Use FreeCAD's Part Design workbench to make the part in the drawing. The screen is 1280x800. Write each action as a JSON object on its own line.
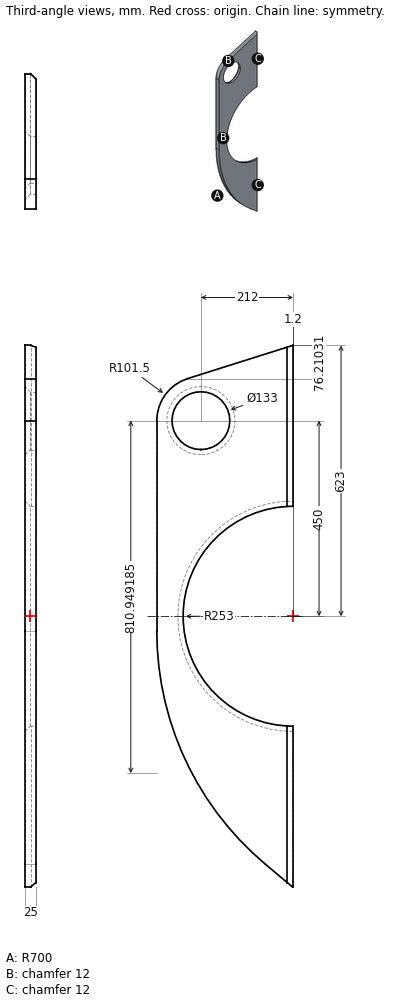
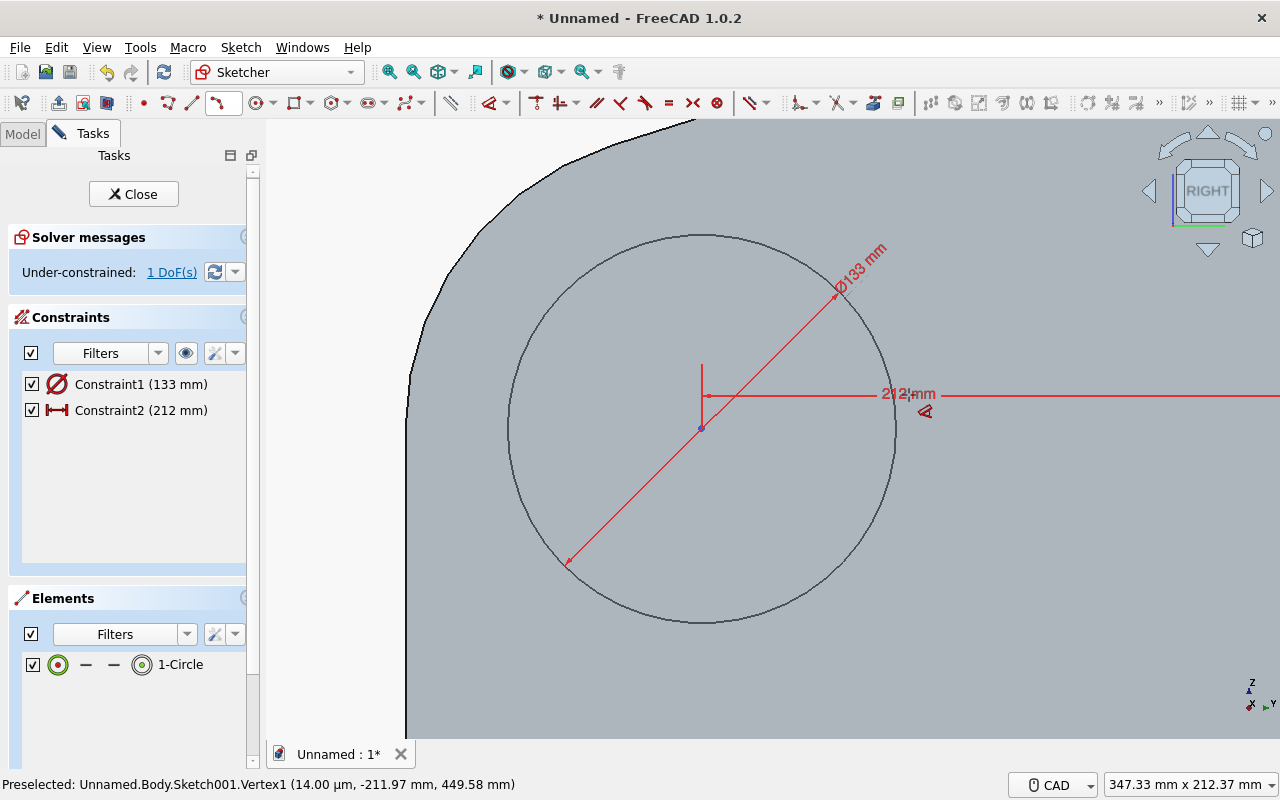
{"action": "left_click", "coordinate": [702, 429]}
{"action": "left_click", "coordinate": [668, 570]}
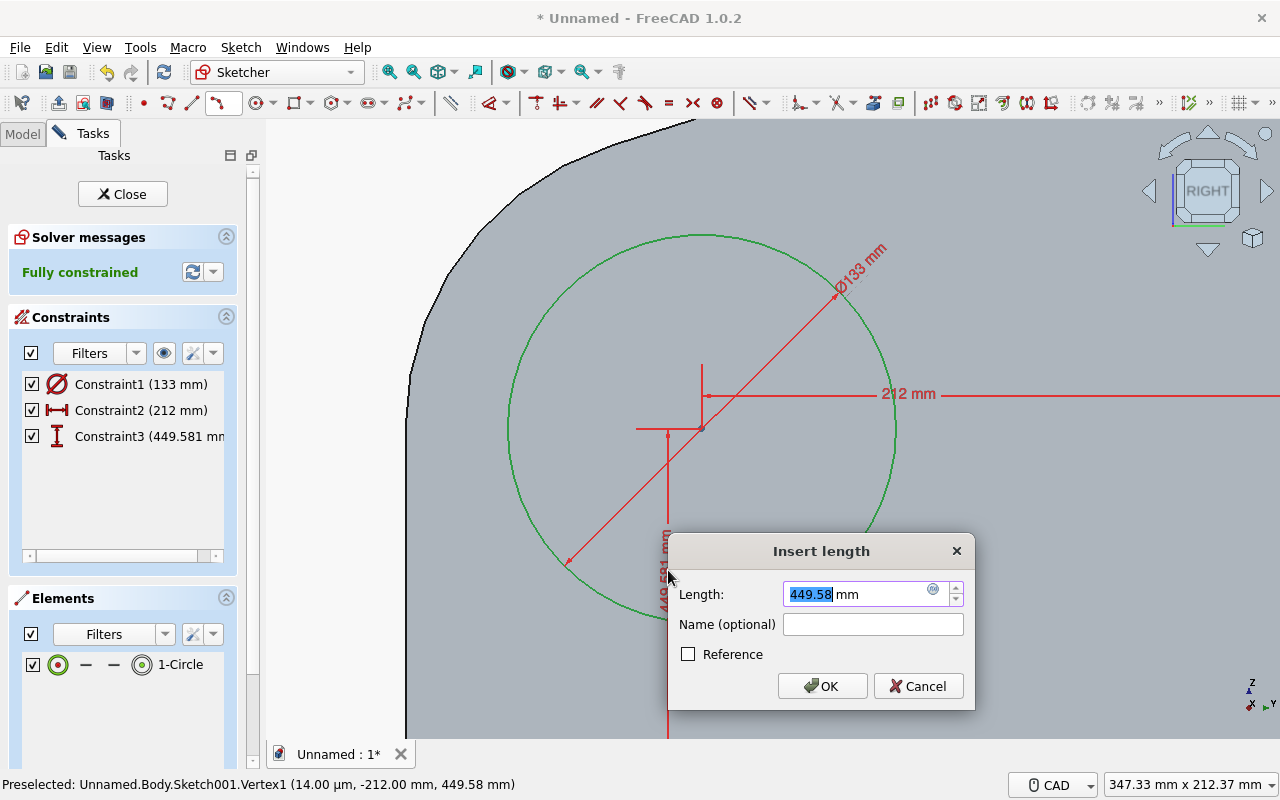
{"action": "type", "text": "450"}
{"action": "key", "text": "Return"}
{"action": "key", "text": "Escape"}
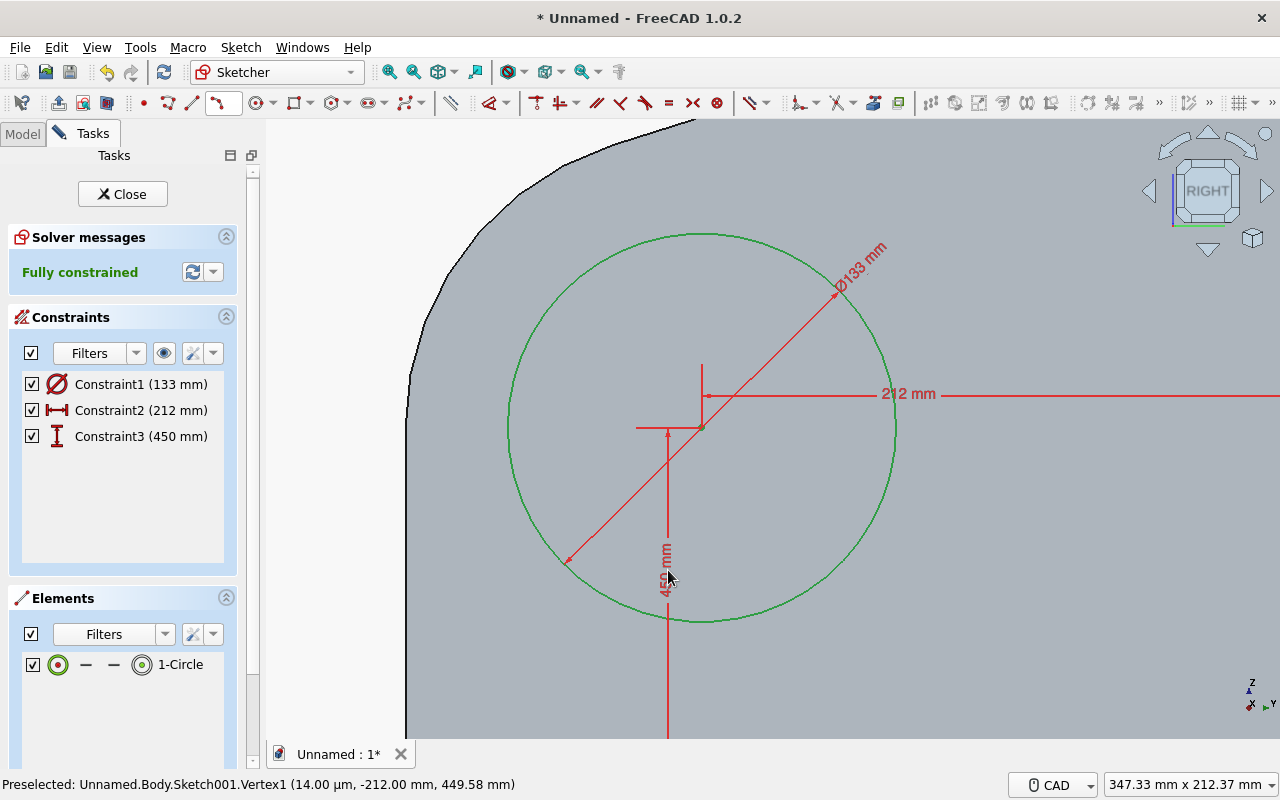
{"action": "left_click", "coordinate": [123, 194]}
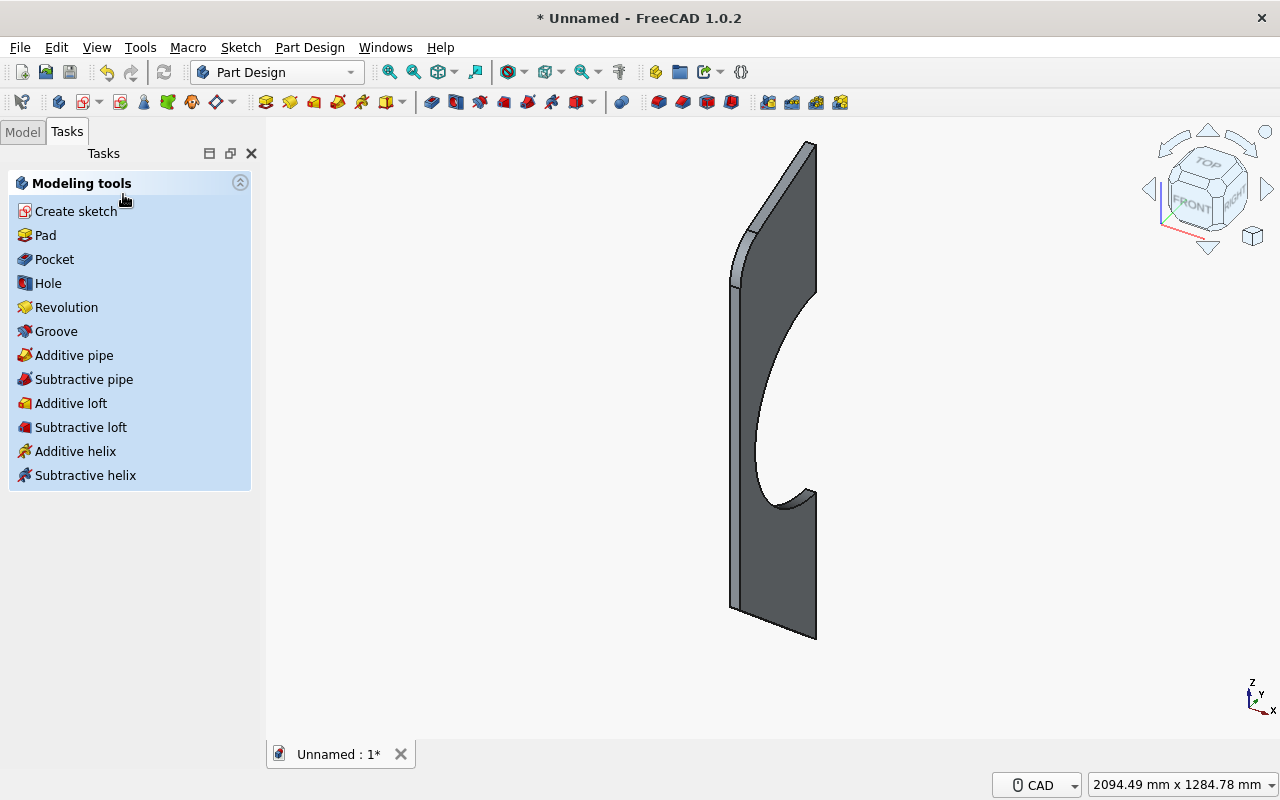
{"action": "left_click", "coordinate": [432, 102]}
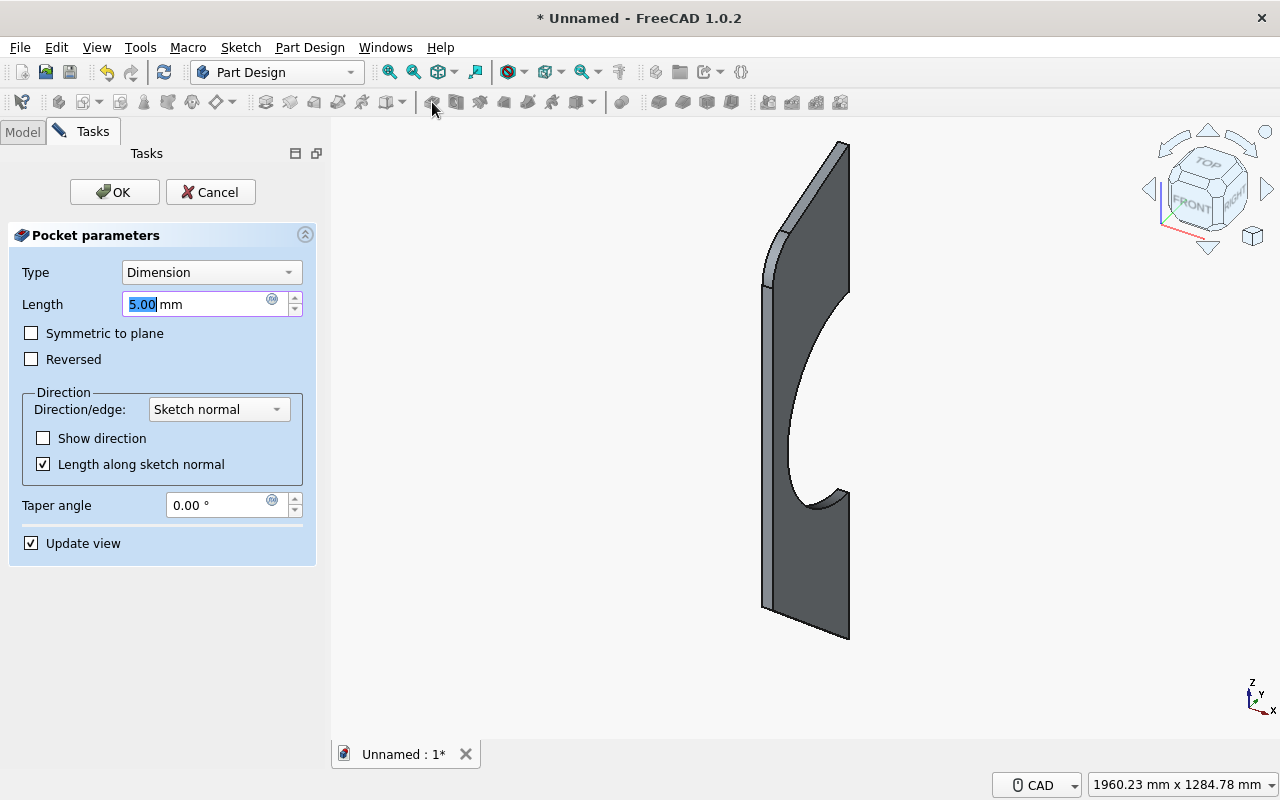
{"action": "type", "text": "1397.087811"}
{"action": "key", "text": "Tab"}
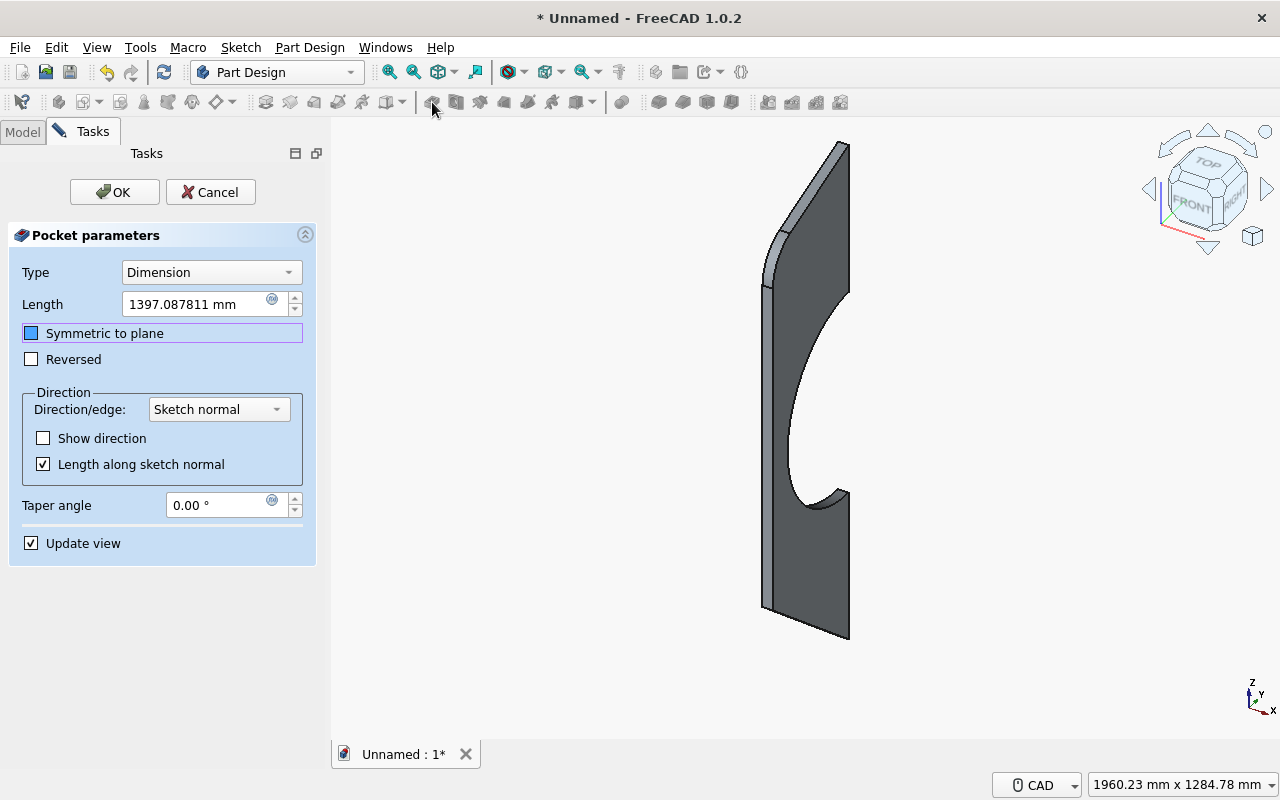
{"action": "left_click", "coordinate": [30, 333]}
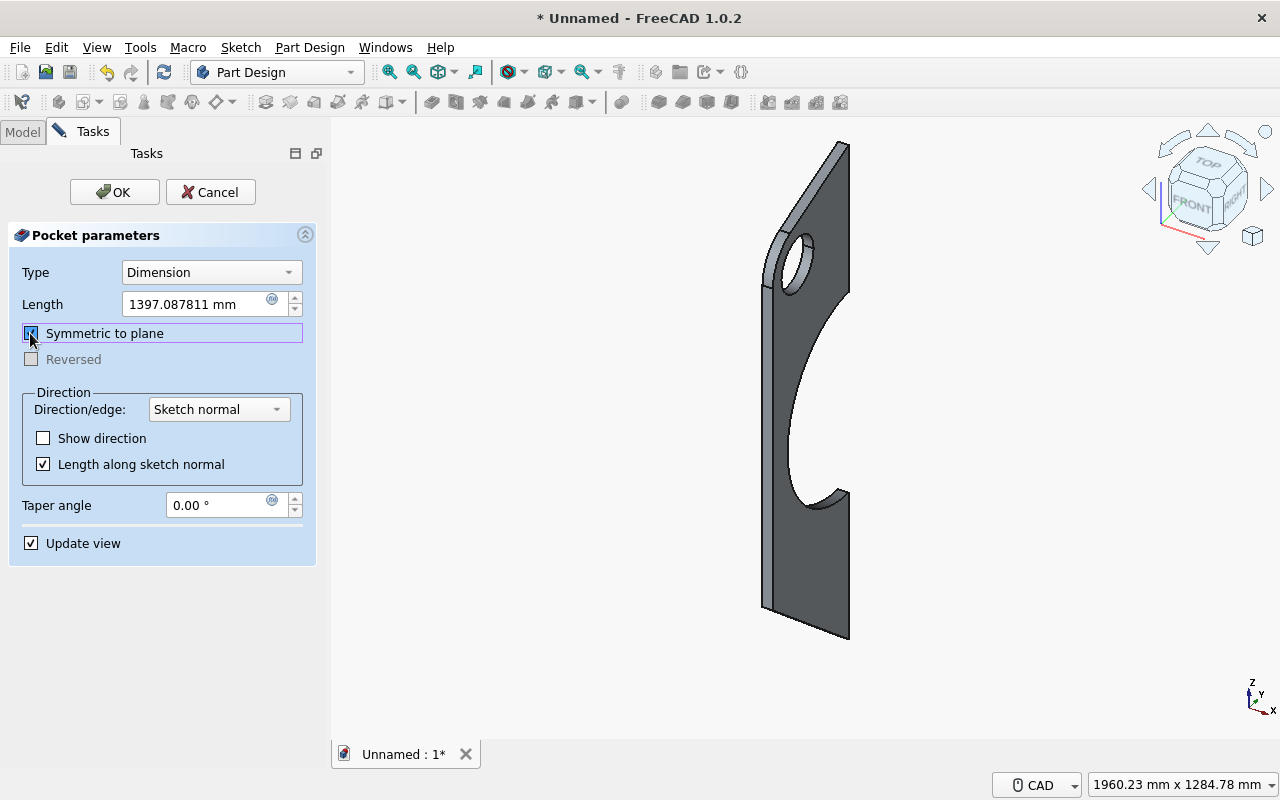
{"action": "left_click", "coordinate": [115, 192]}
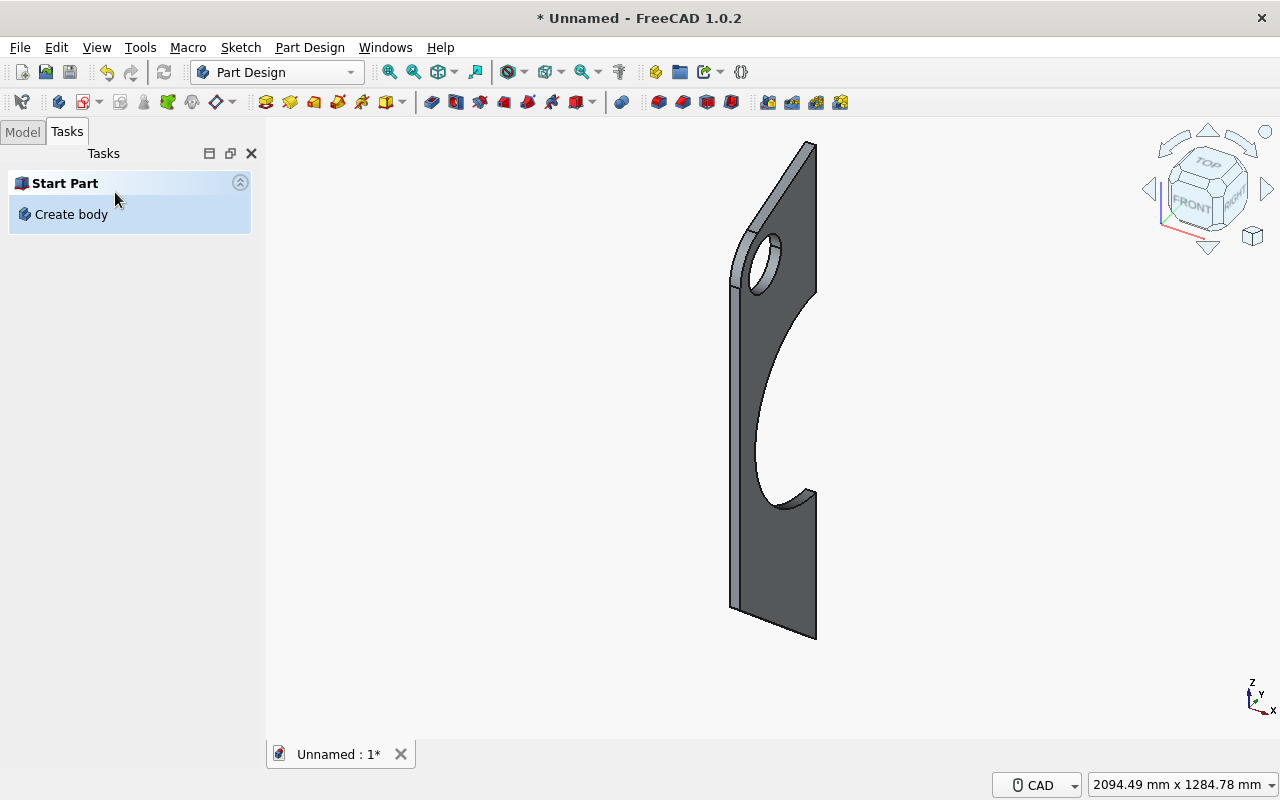
{"action": "scroll", "coordinate": [735, 608], "scroll_direction": "up", "scroll_amount": 6}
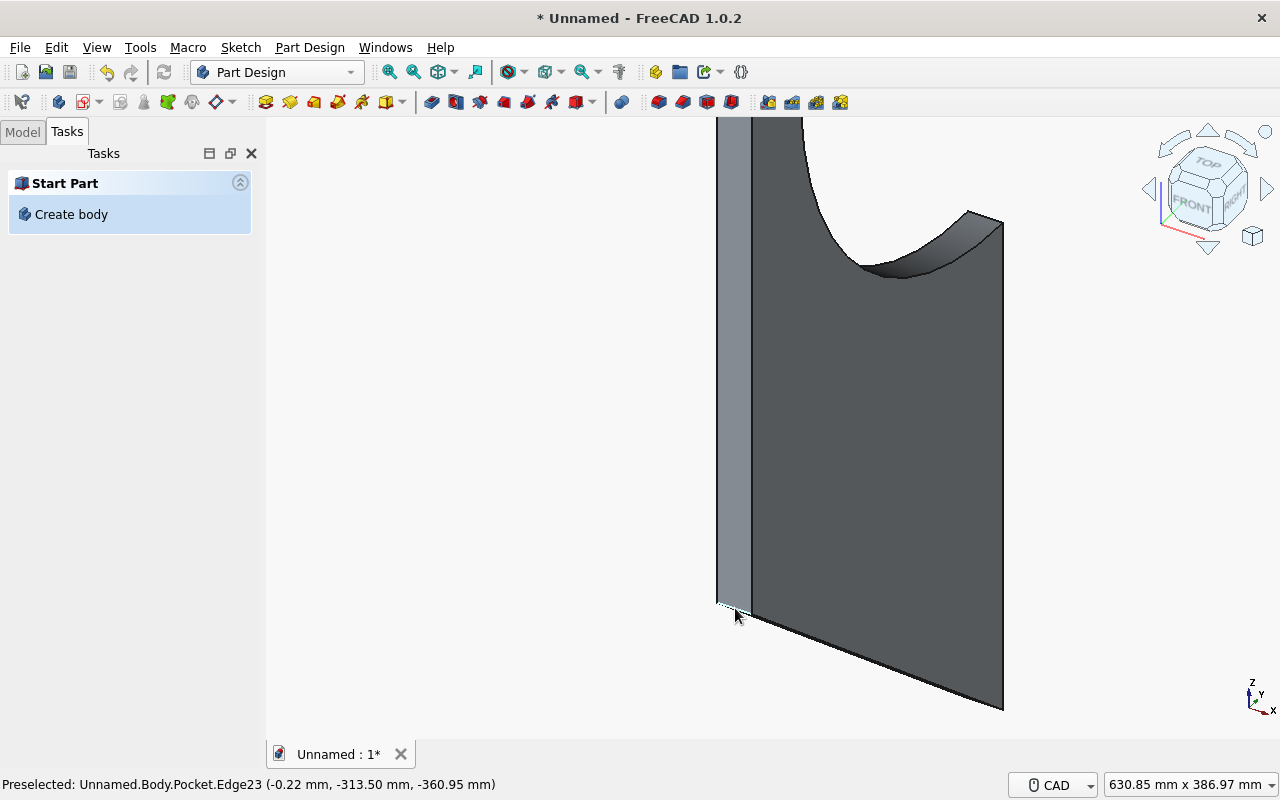
{"action": "left_click", "coordinate": [390, 72]}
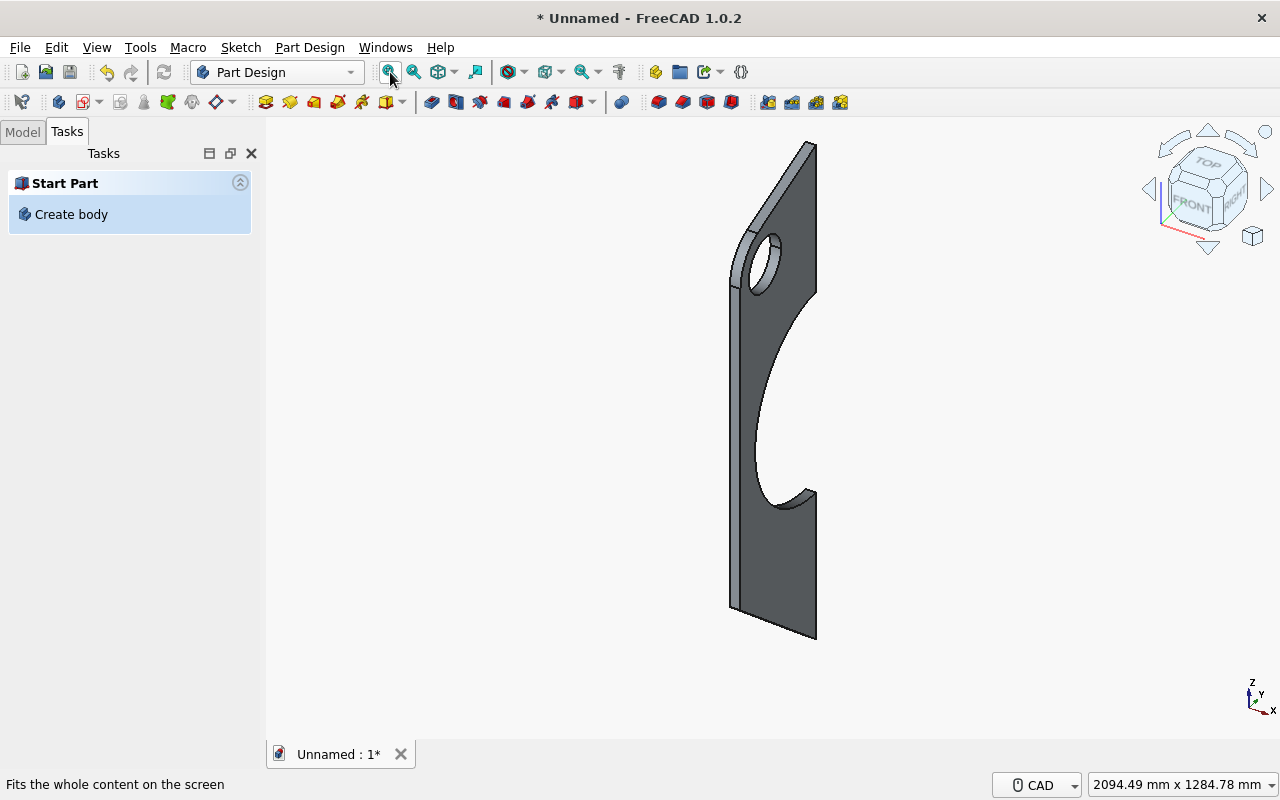
{"action": "key", "text": "0"}